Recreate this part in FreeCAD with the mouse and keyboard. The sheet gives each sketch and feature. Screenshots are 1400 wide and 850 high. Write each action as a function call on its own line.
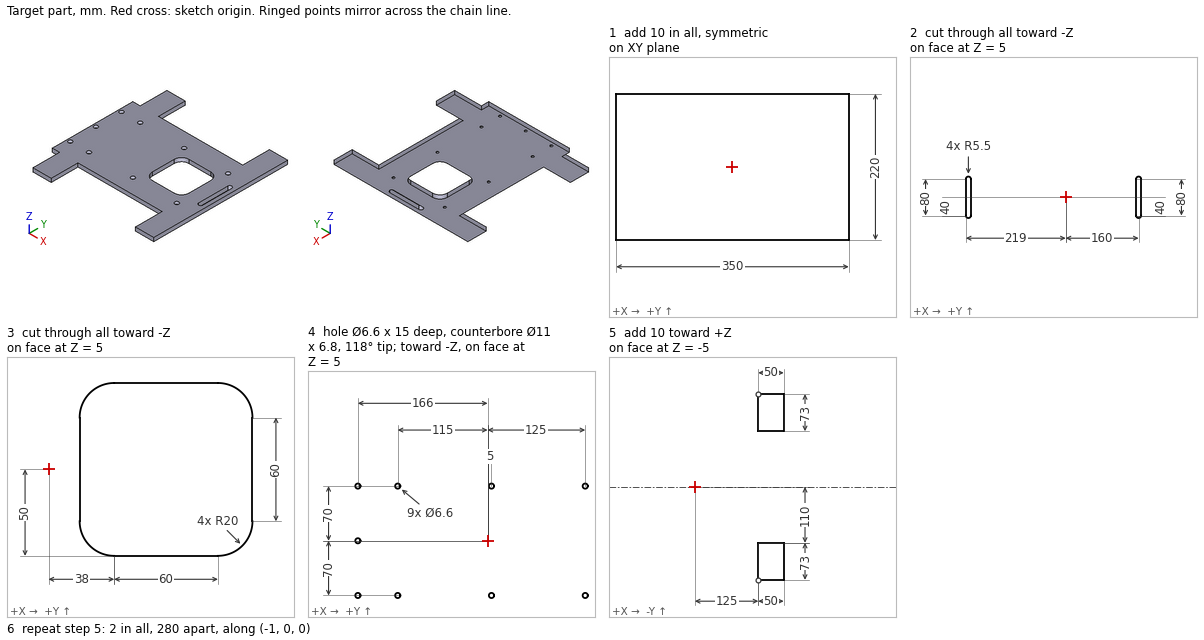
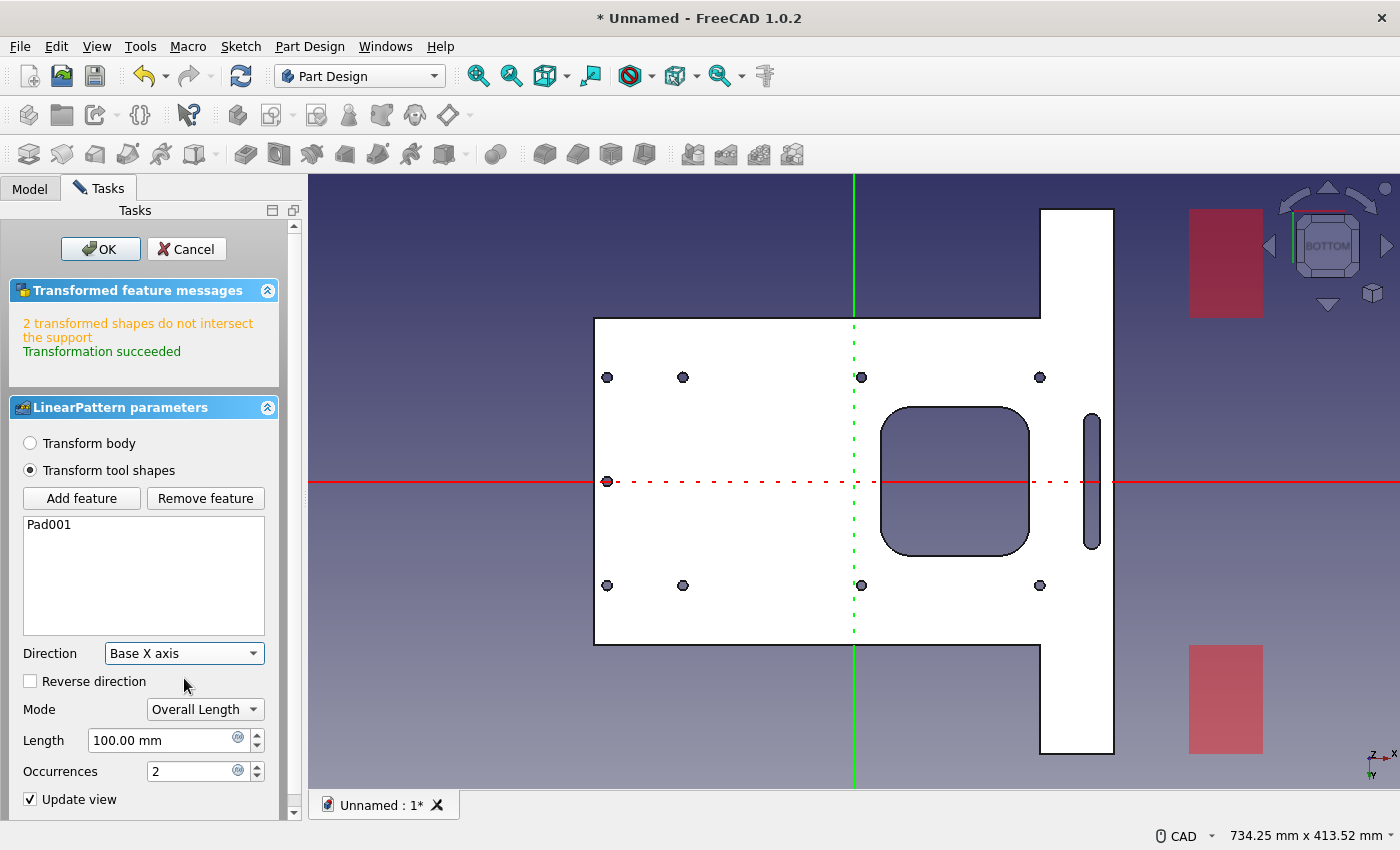
click(206, 710)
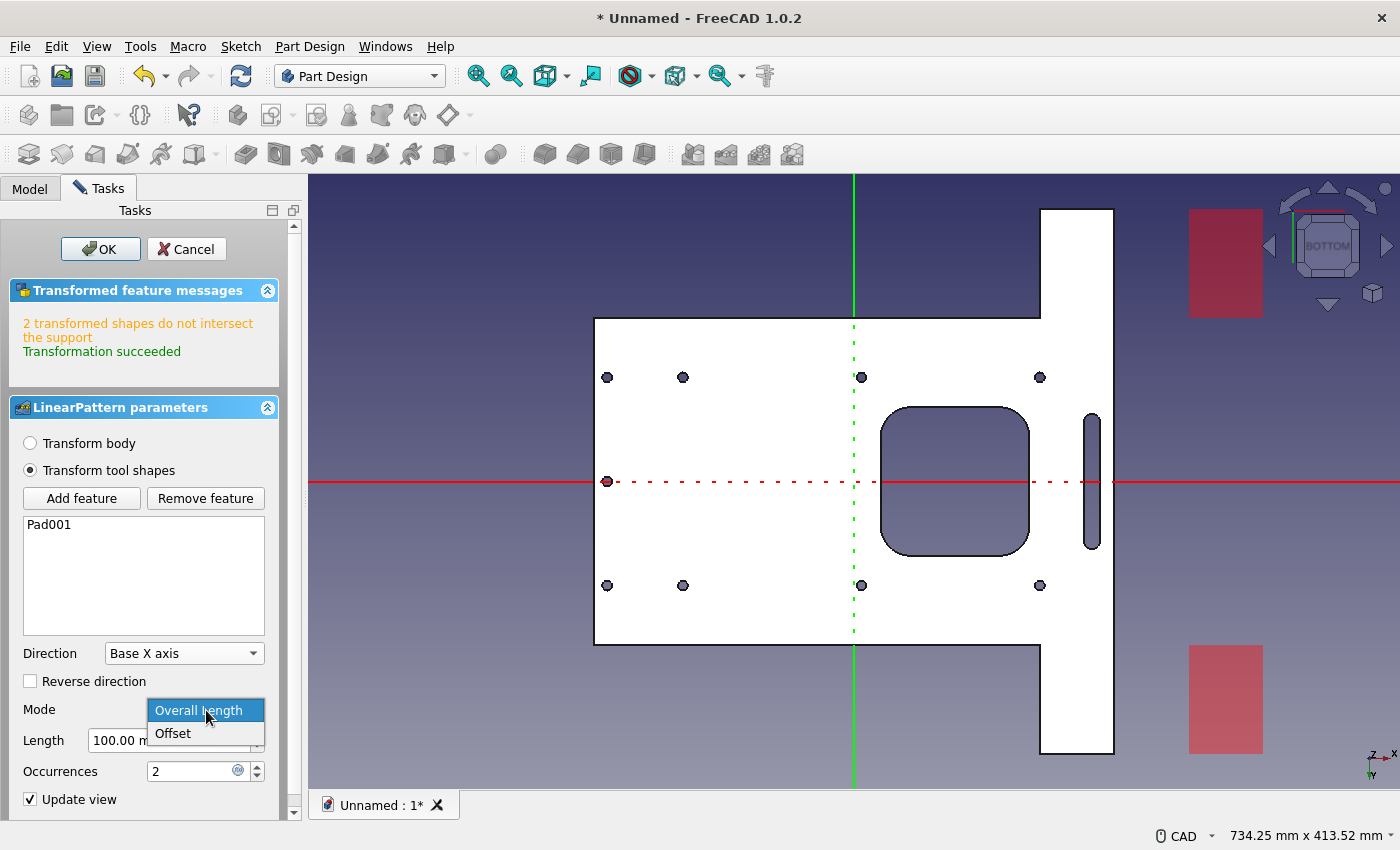
click(204, 734)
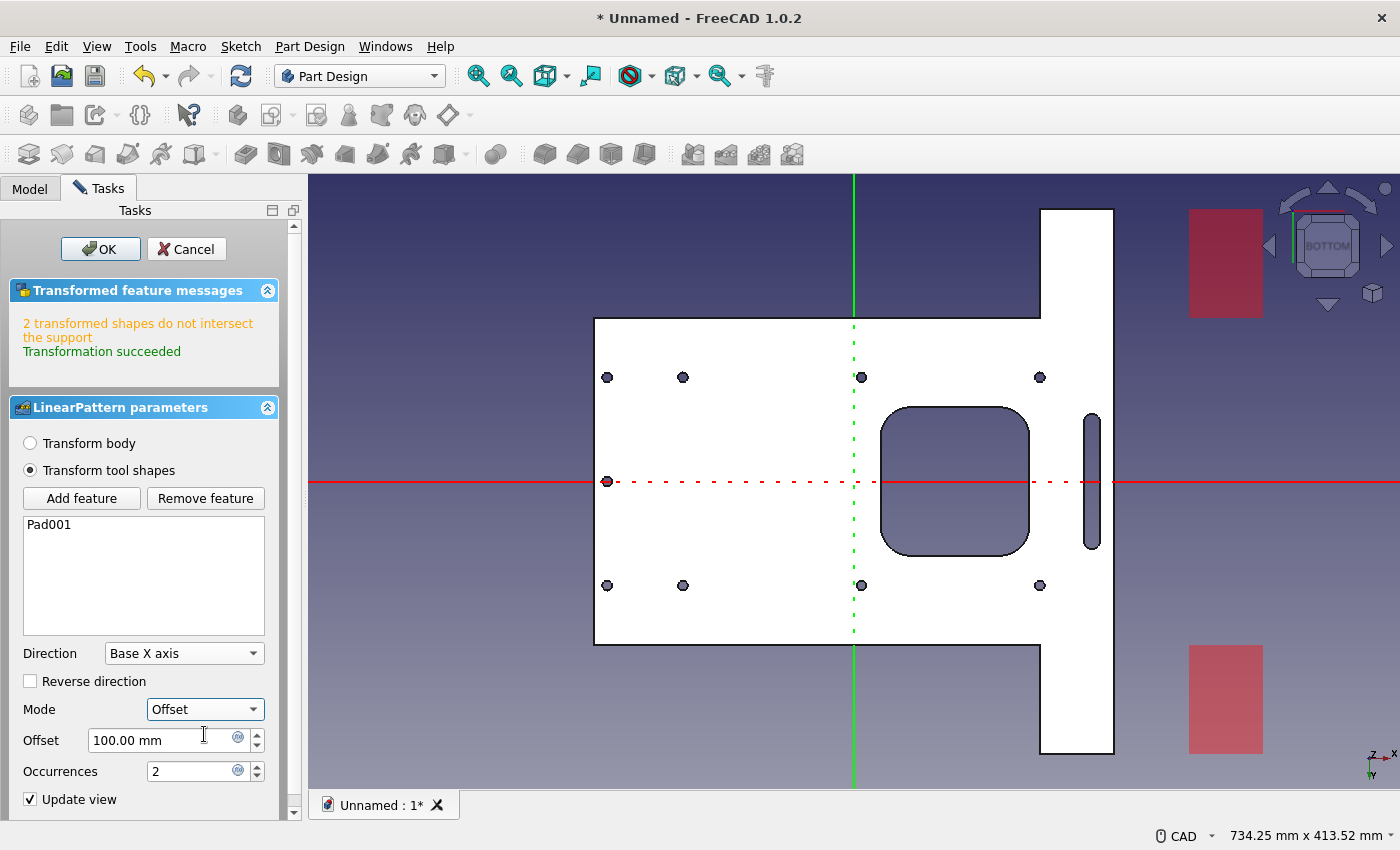
triple_click(170, 740)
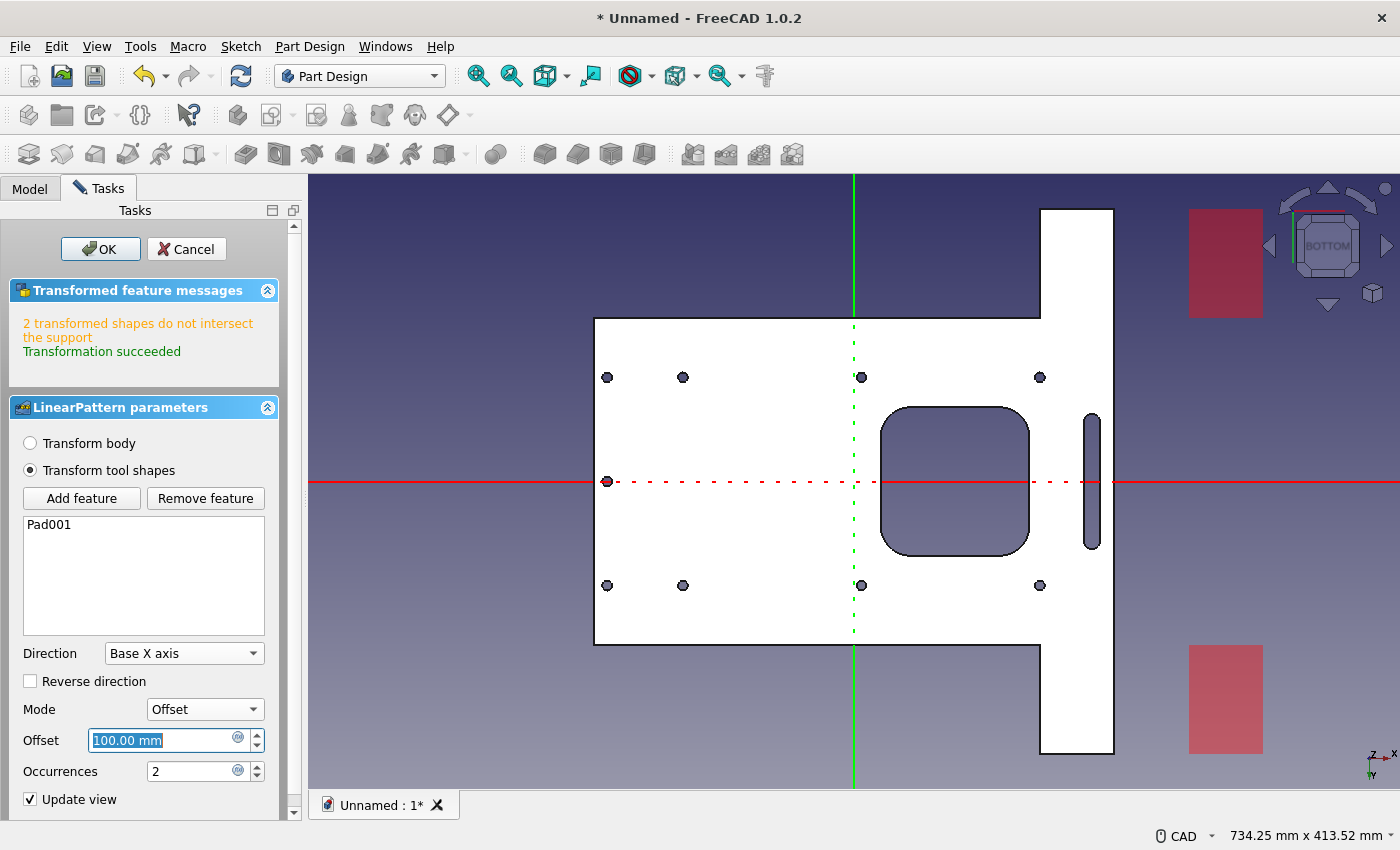
text(280)
key(Tab)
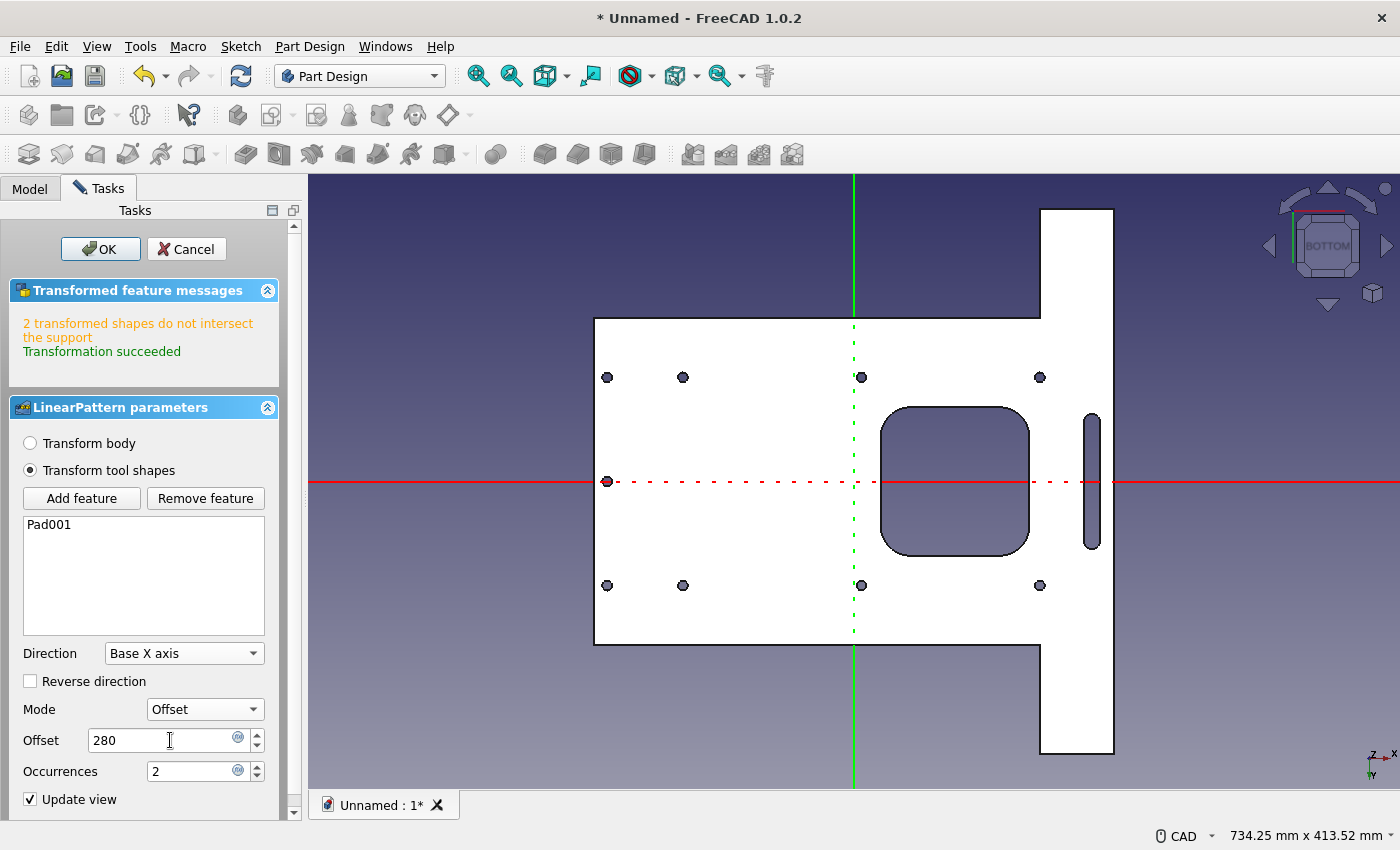
triple_click(199, 772)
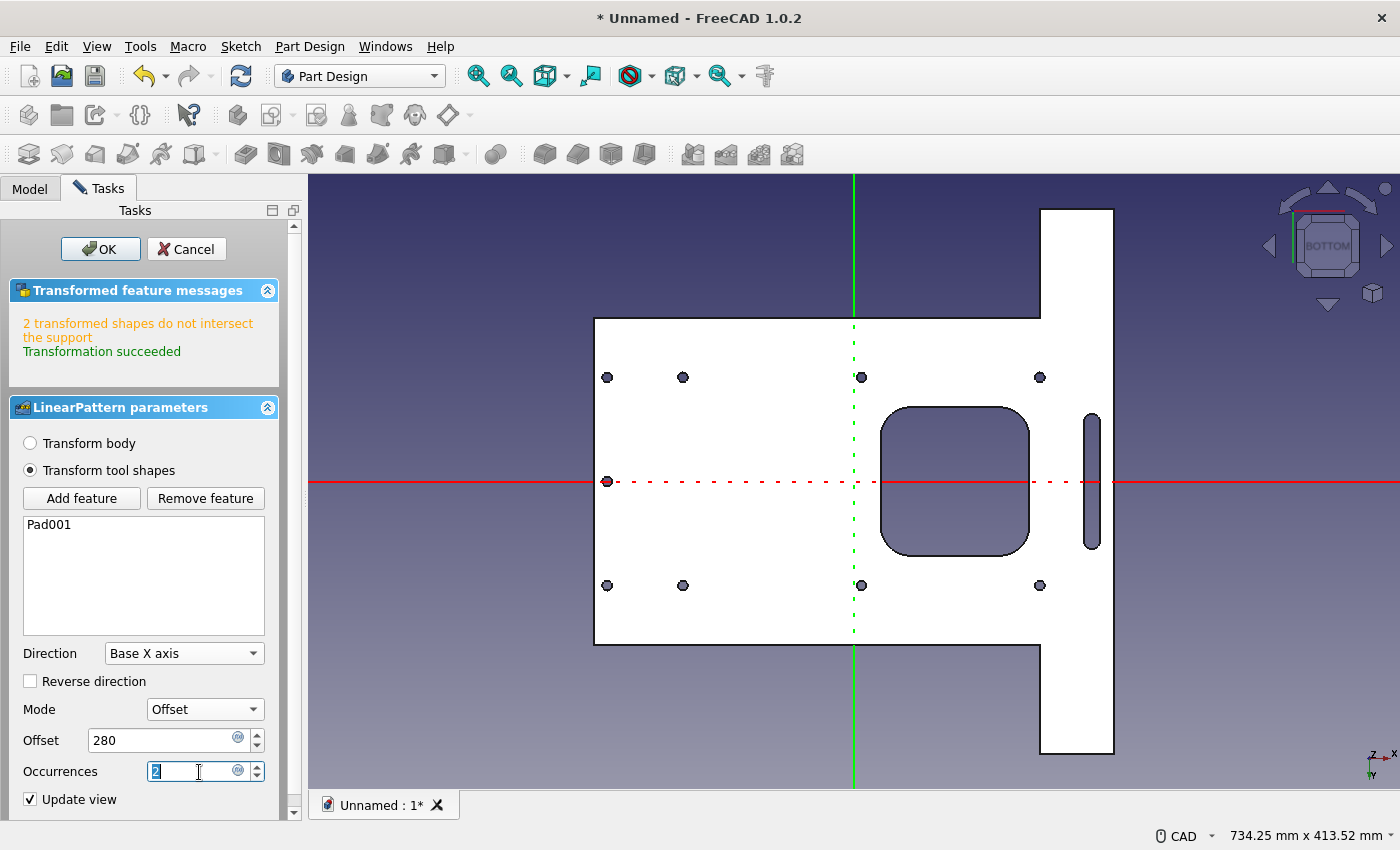
text(2)
key(Tab)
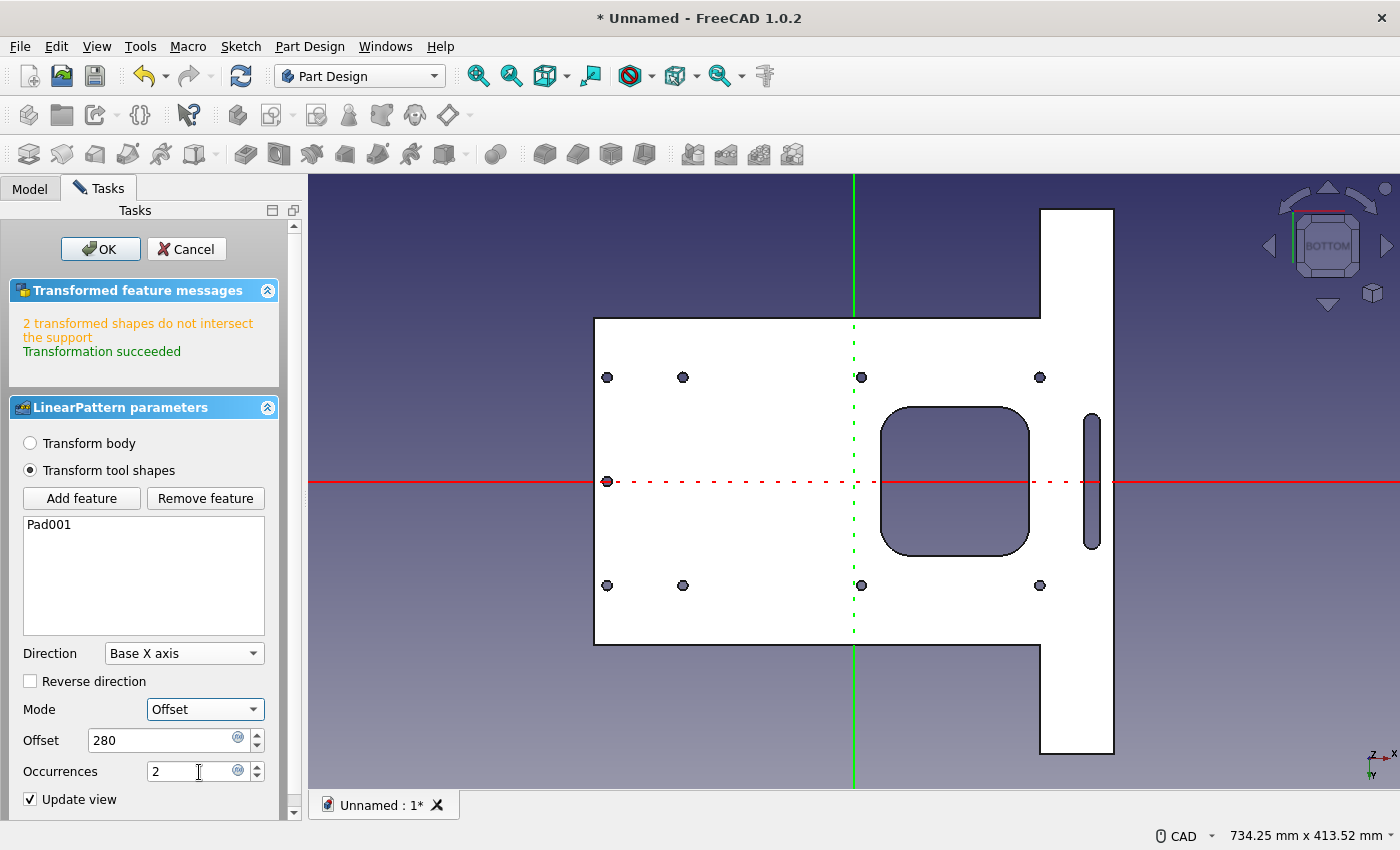
click(31, 681)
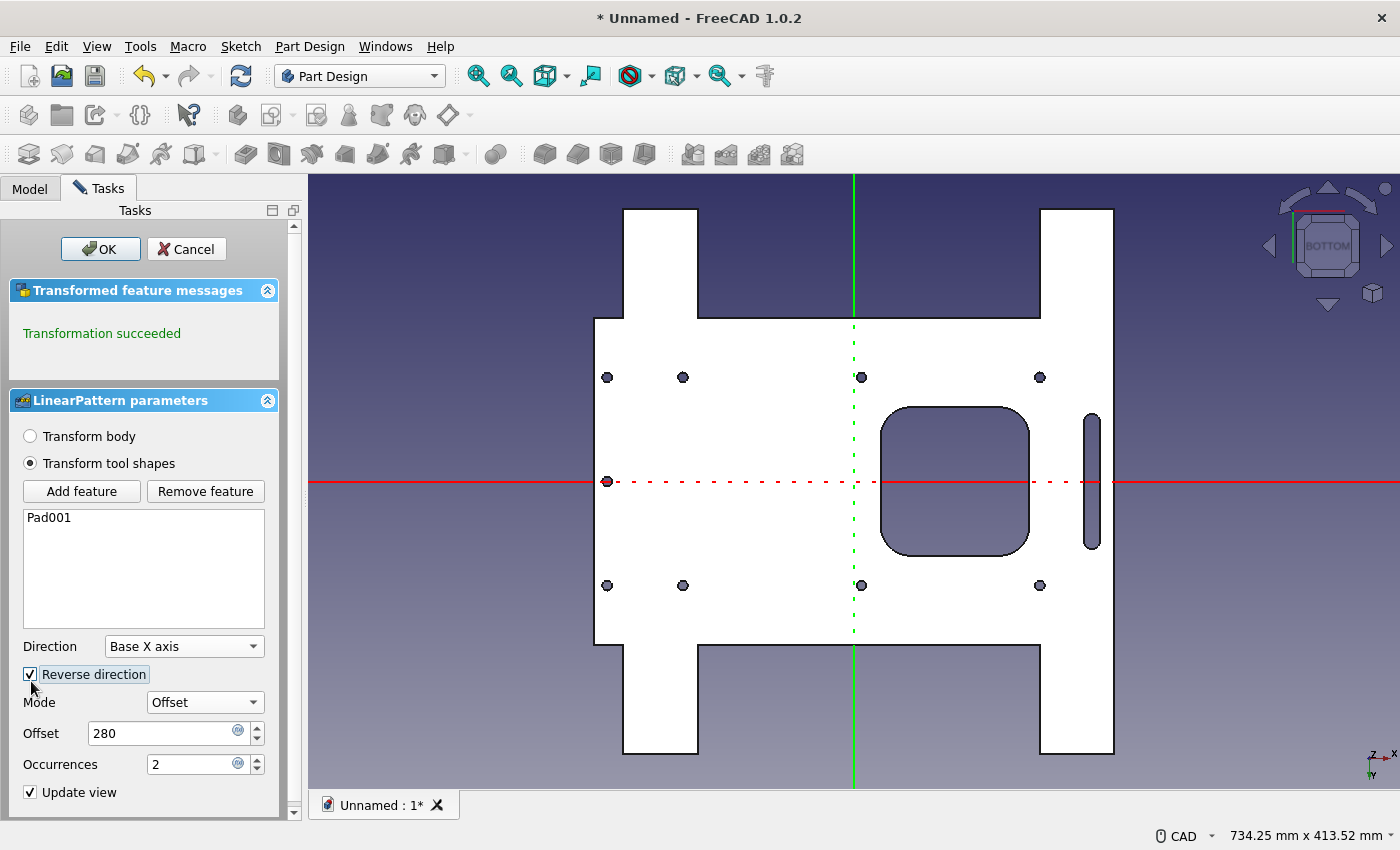
click(101, 249)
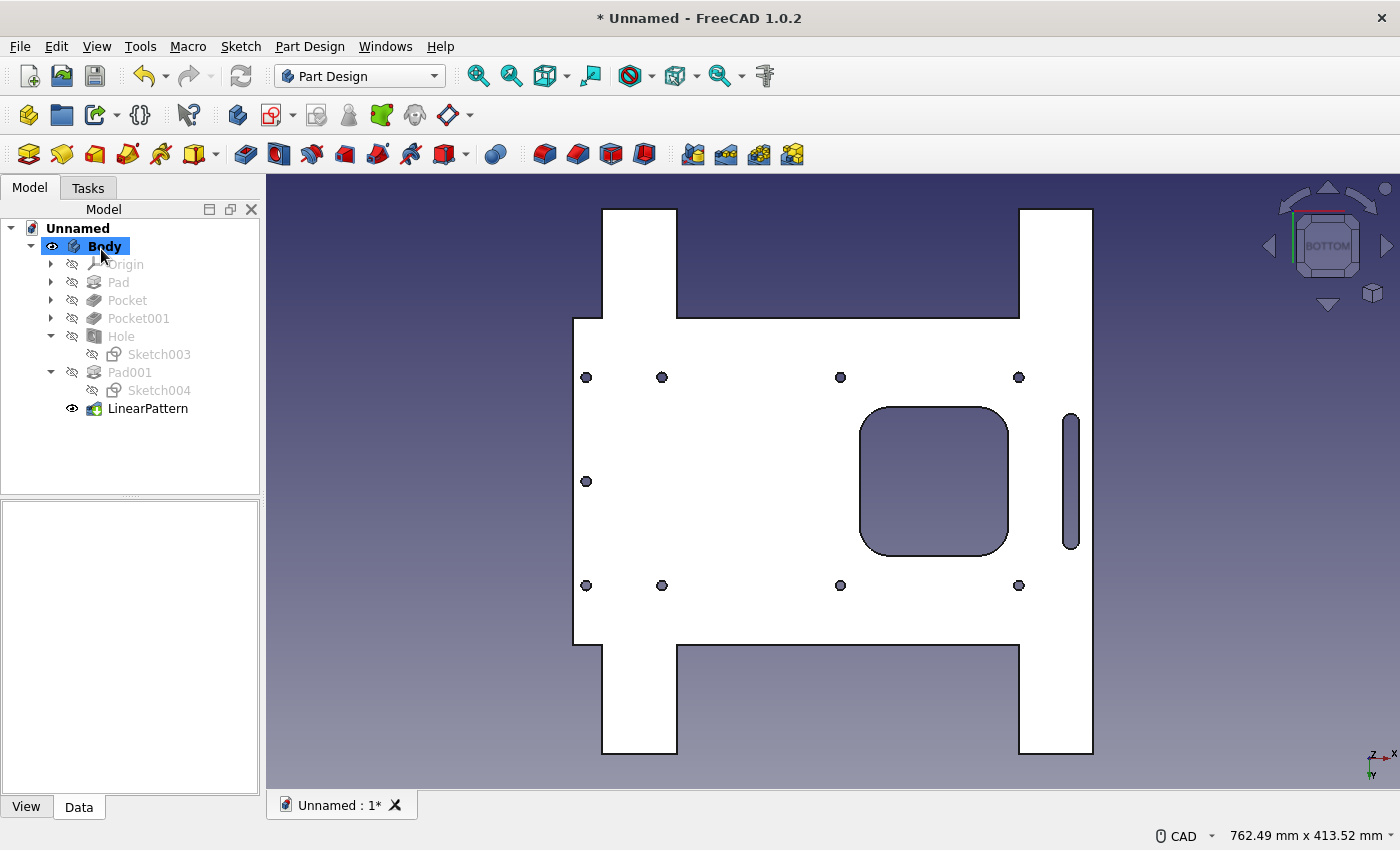
key(0)